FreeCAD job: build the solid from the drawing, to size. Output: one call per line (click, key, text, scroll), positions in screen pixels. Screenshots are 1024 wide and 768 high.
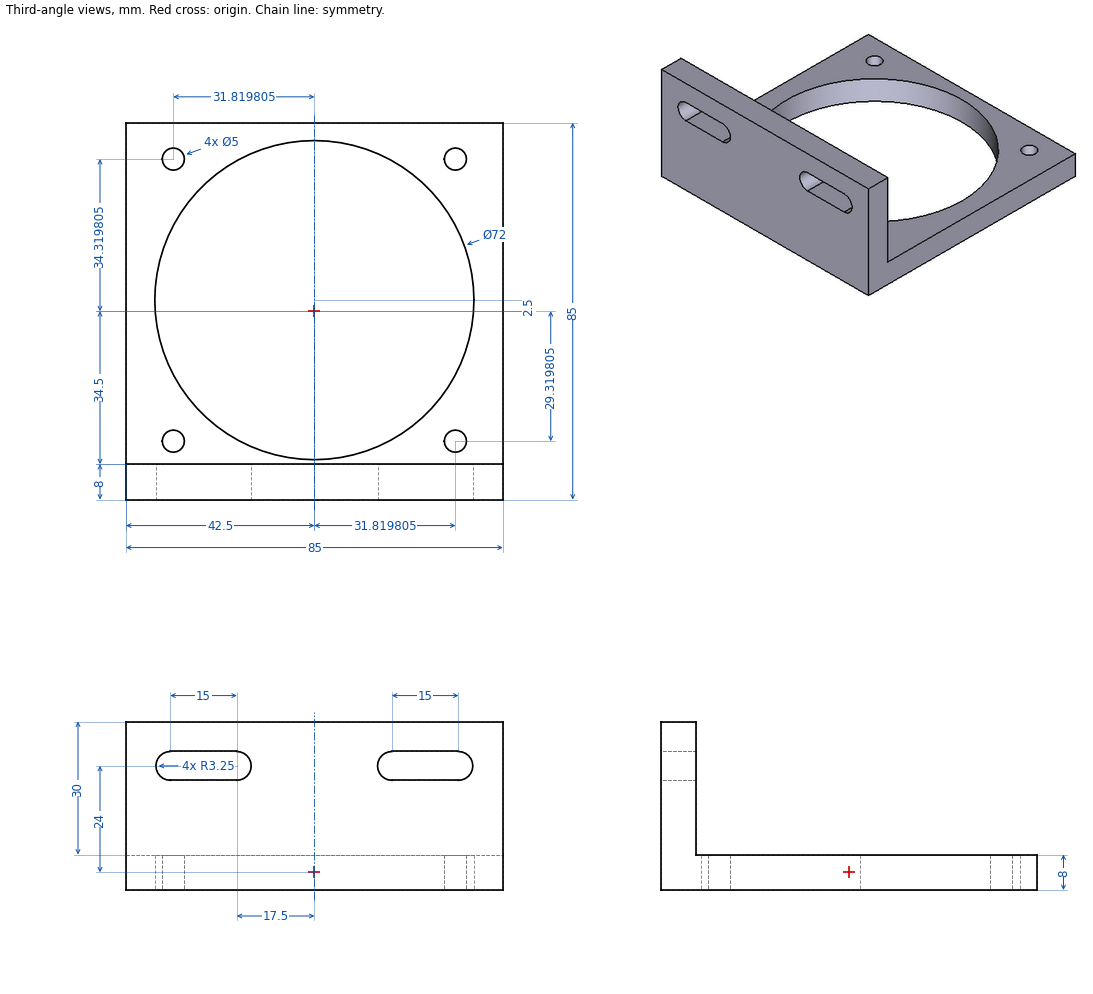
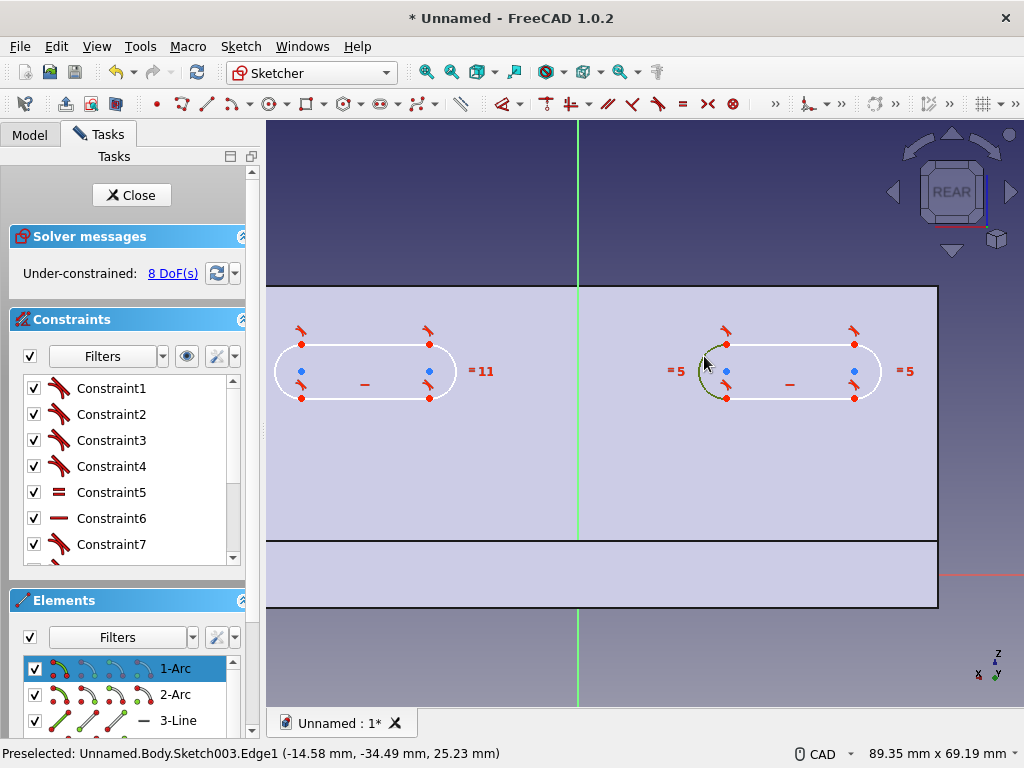
scroll(574, 321, down, 2)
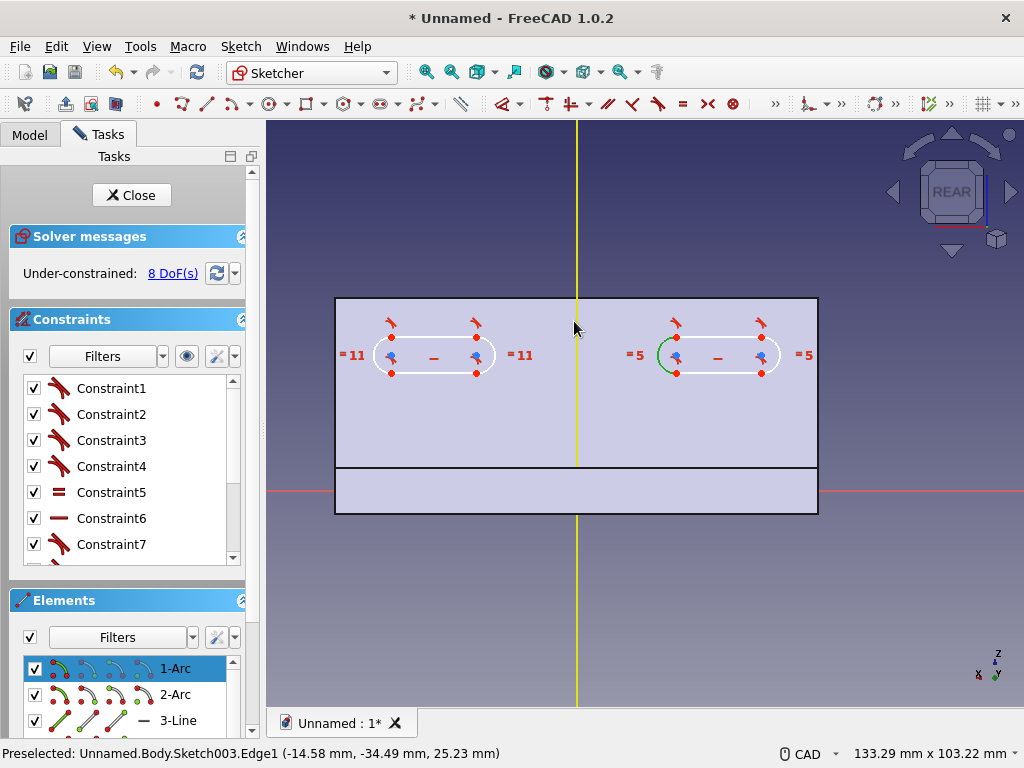
click(377, 345)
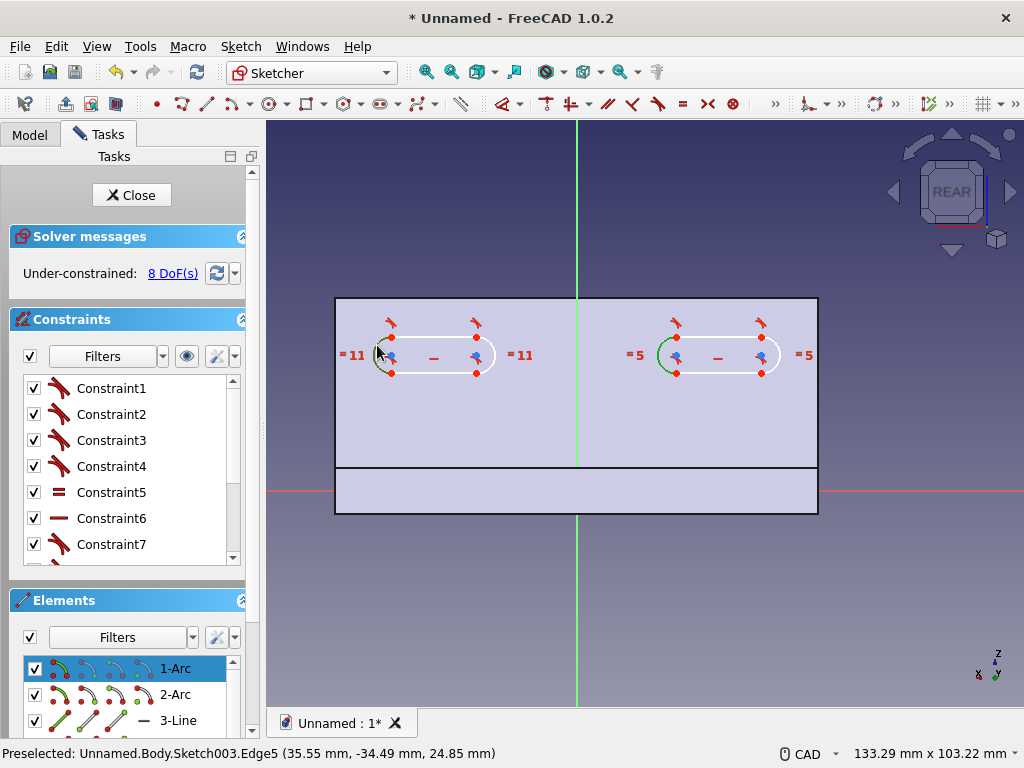
key(e)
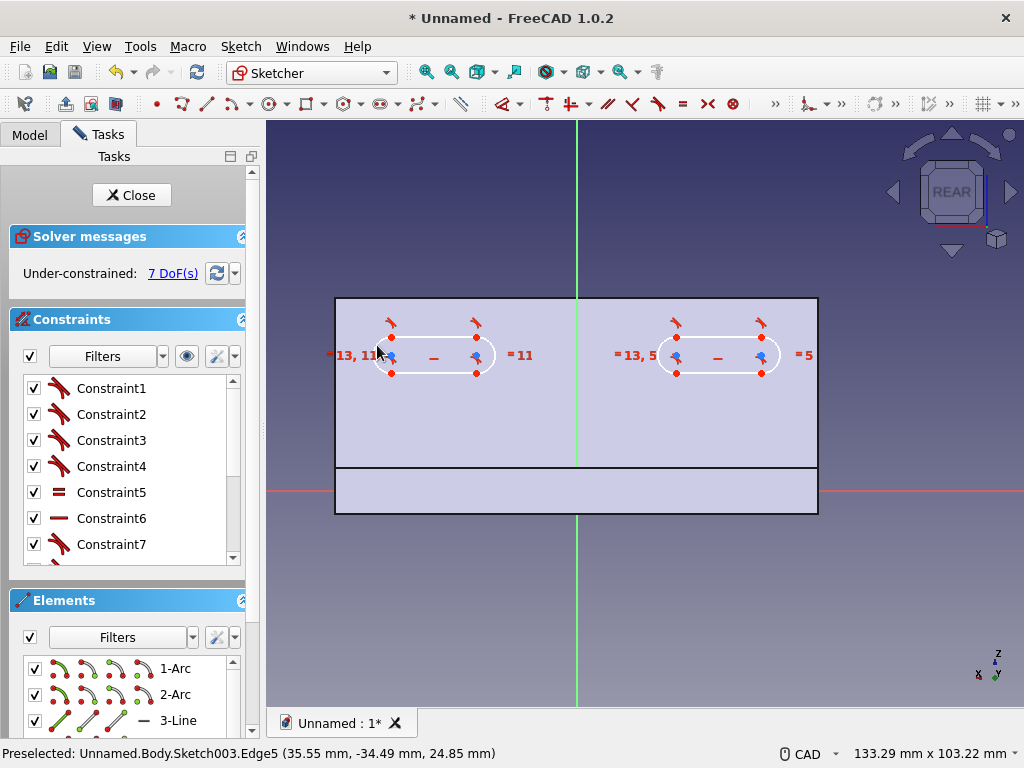
click(762, 355)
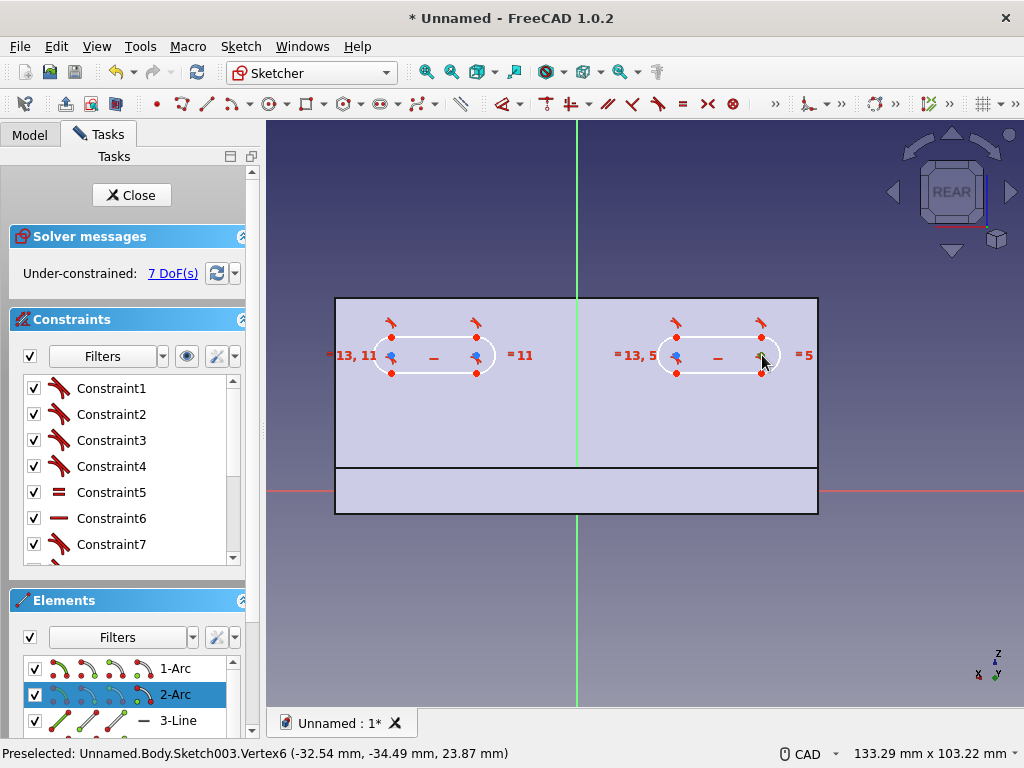
click(392, 355)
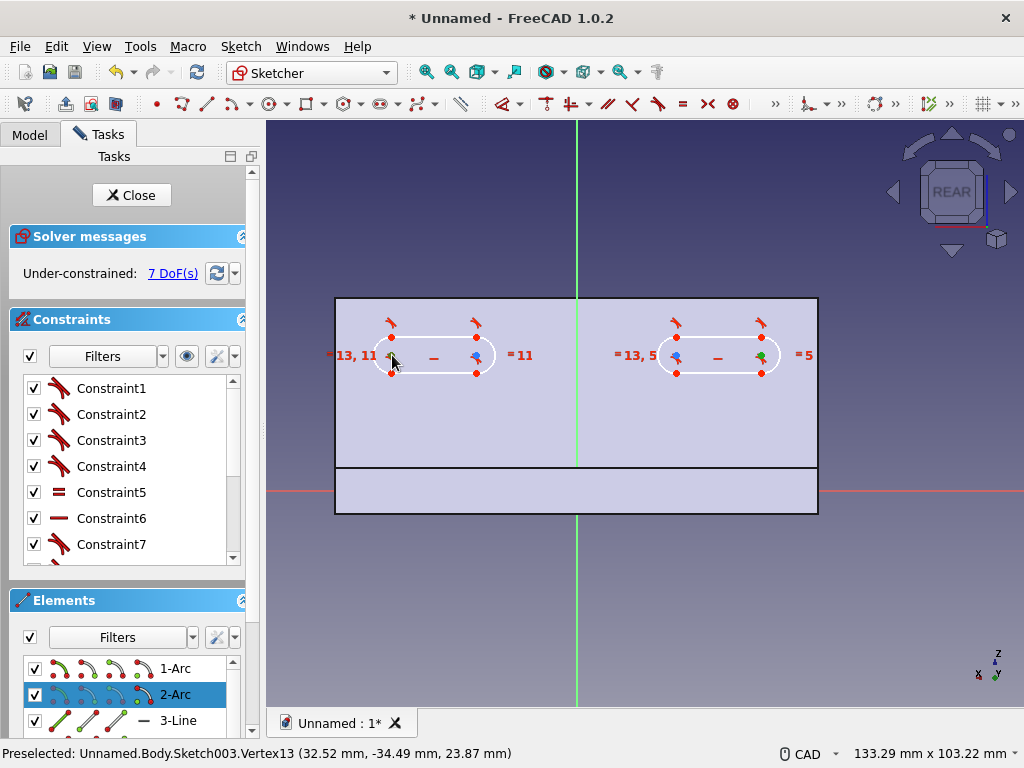
click(577, 641)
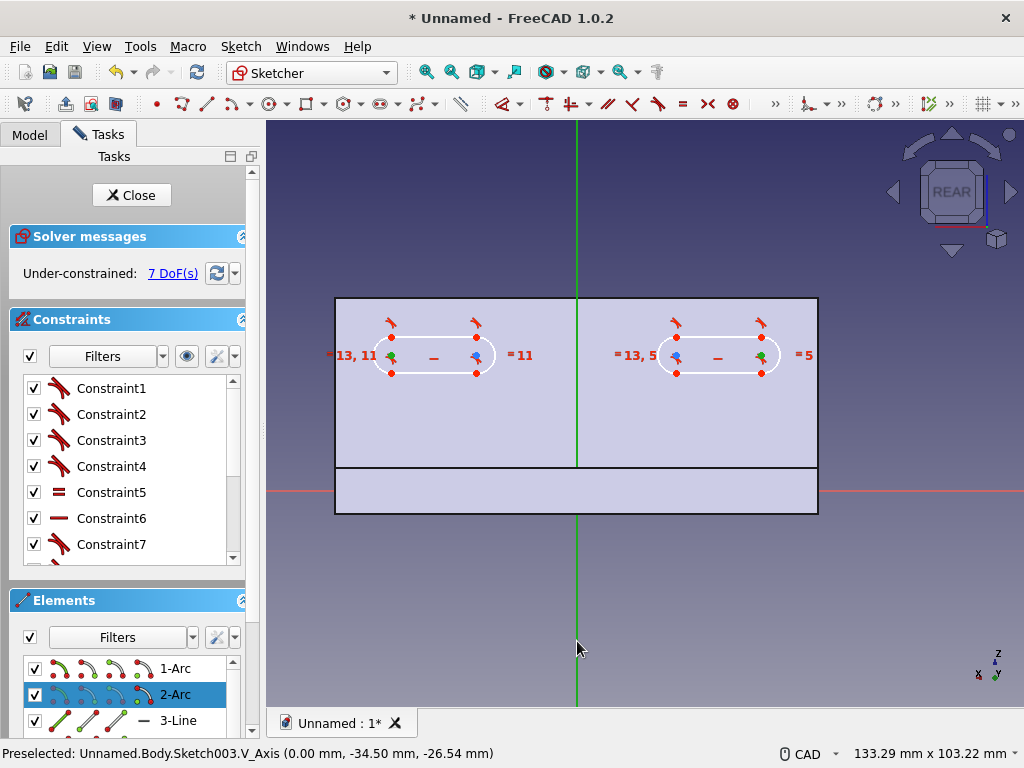
key(s)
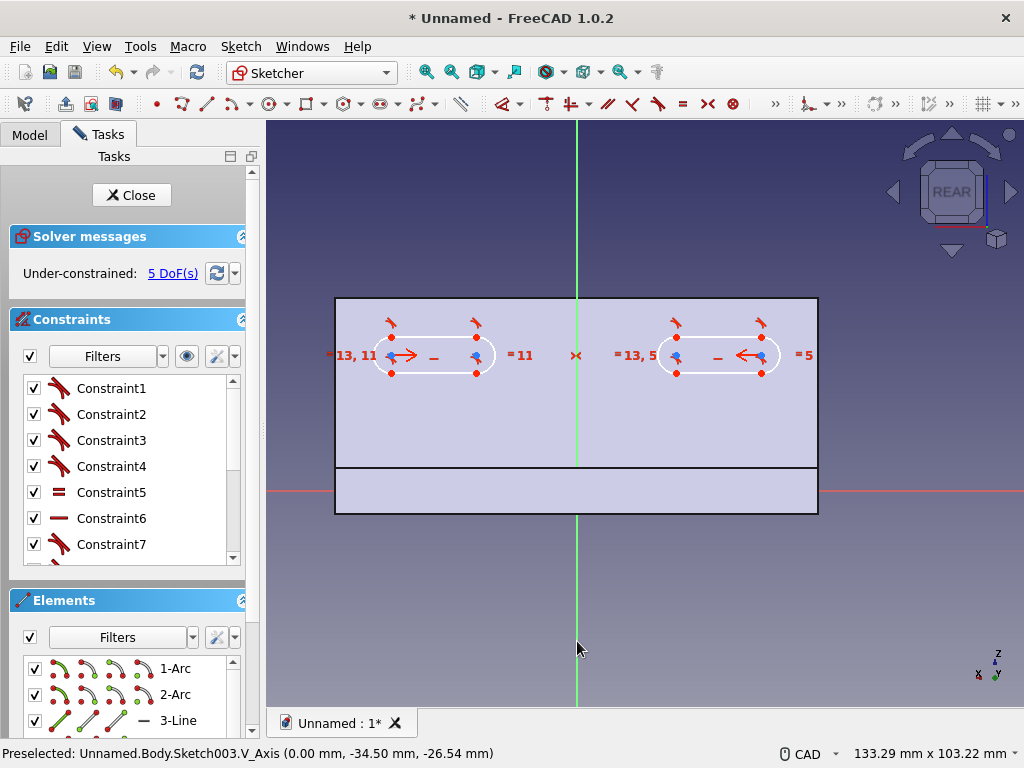
key(d)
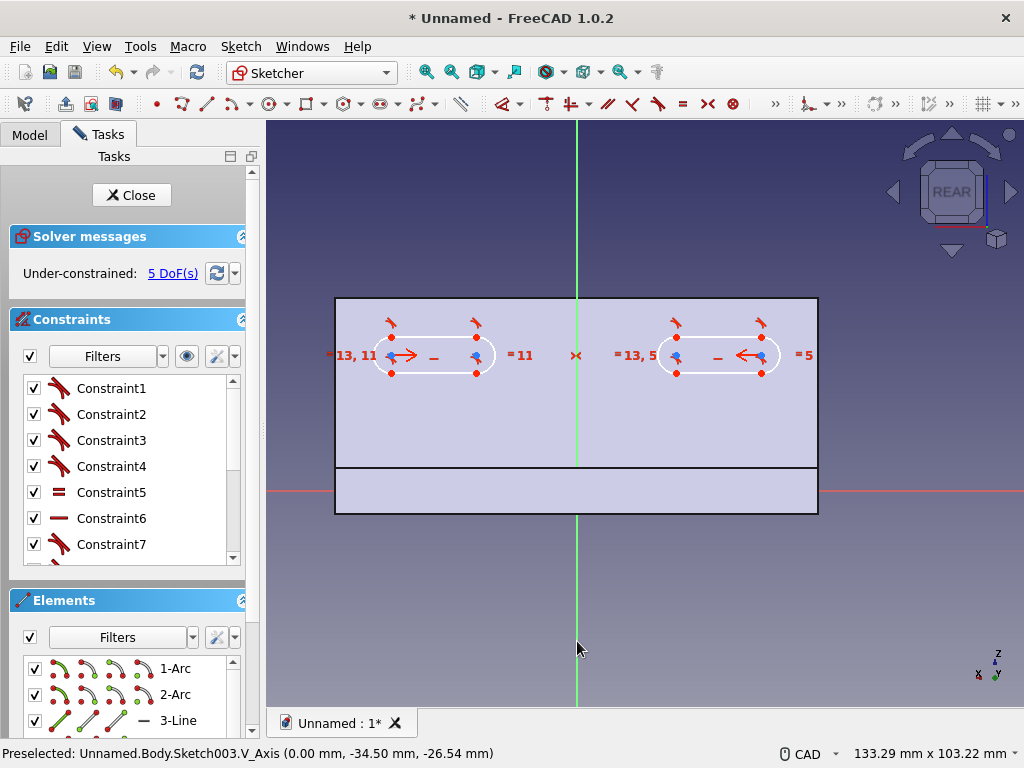
scroll(661, 345, up, 4)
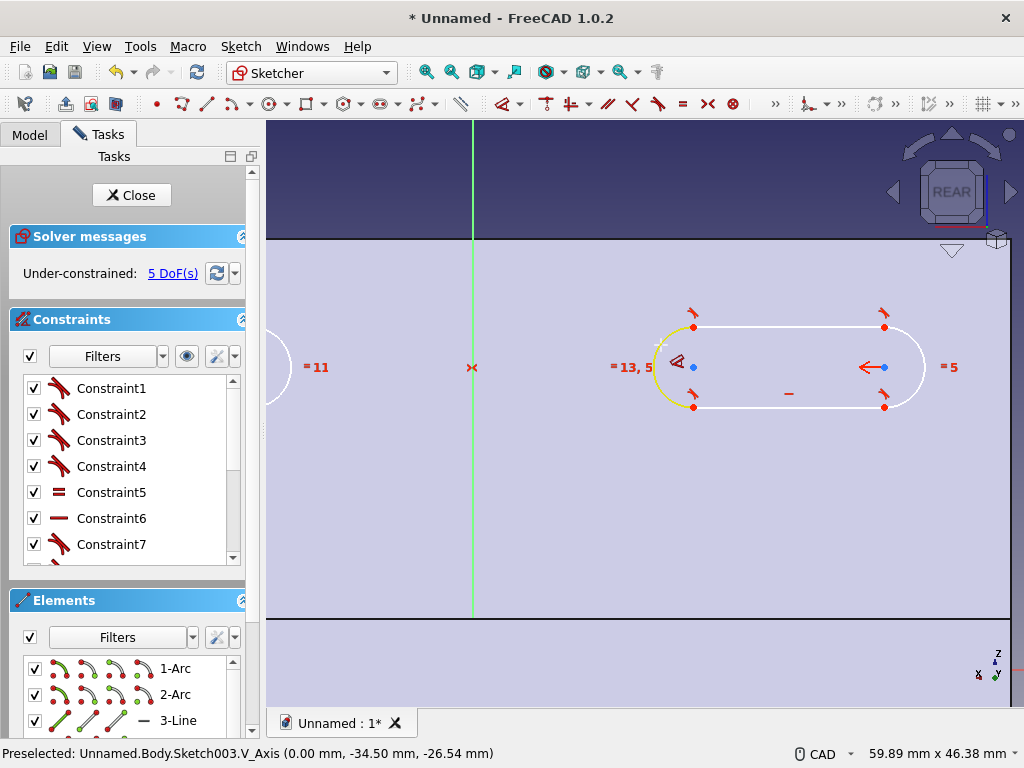
click(661, 344)
click(635, 325)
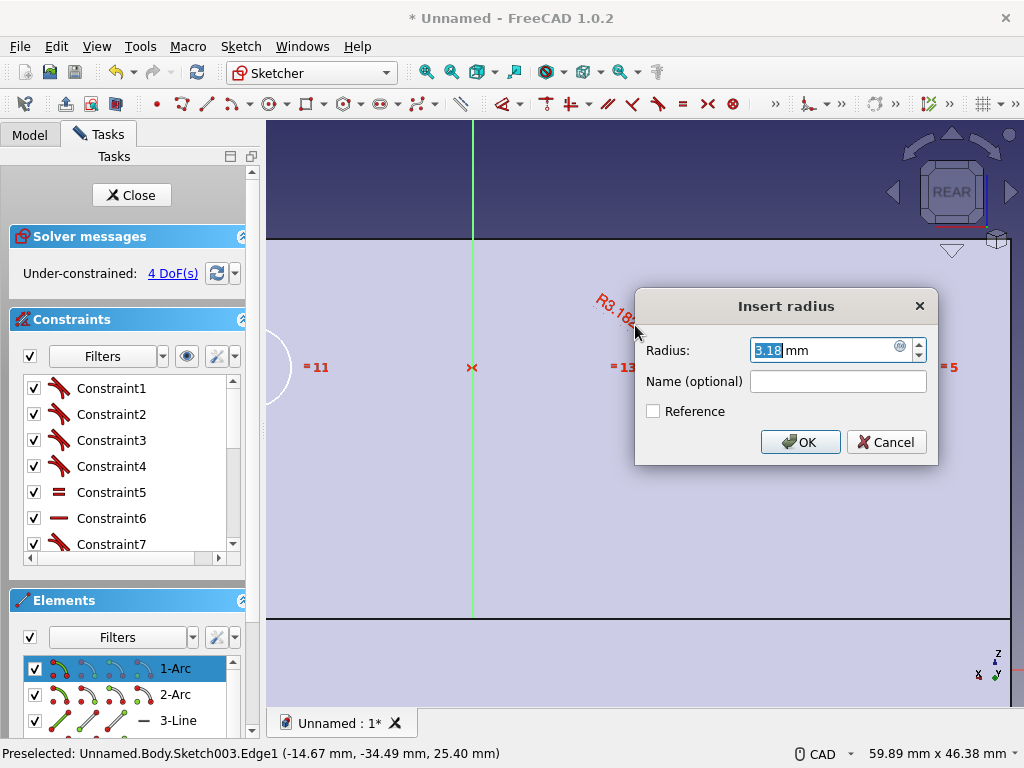
text(3.25)
key(Return)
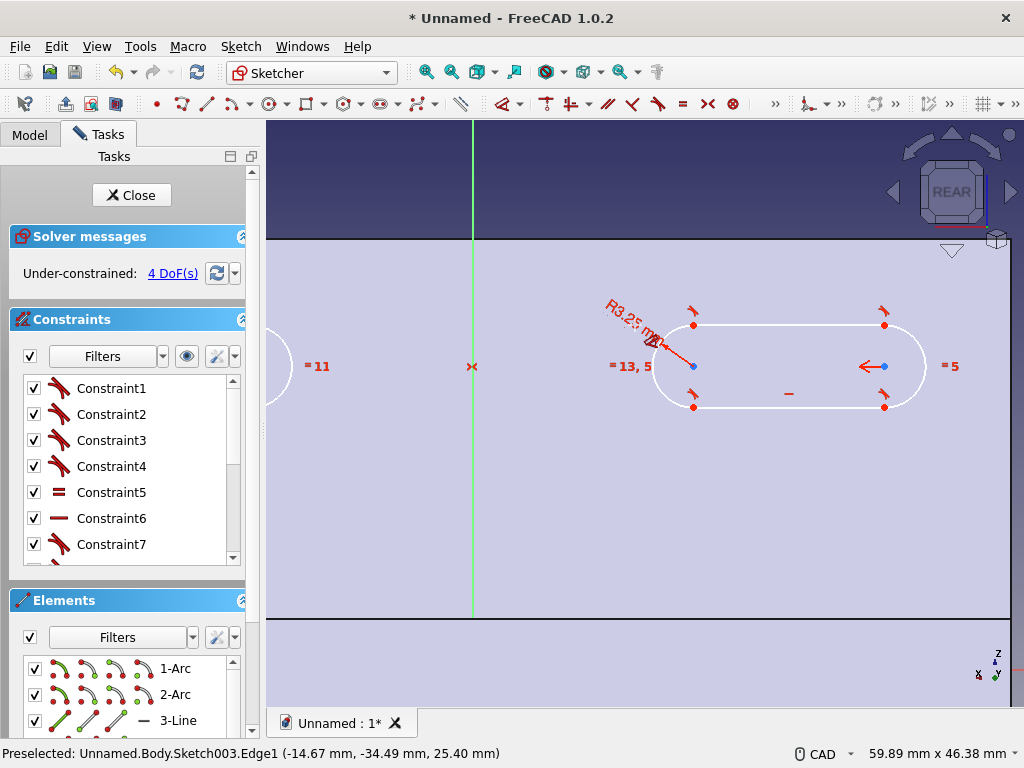
click(751, 325)
click(776, 291)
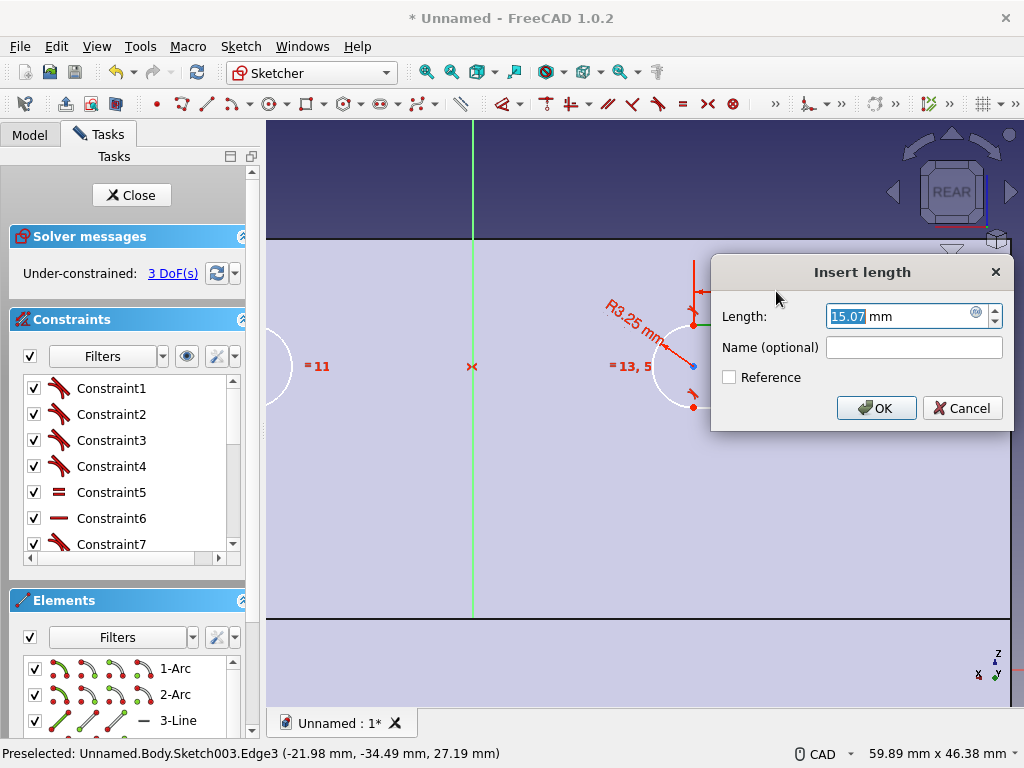
text(15)
key(Return)